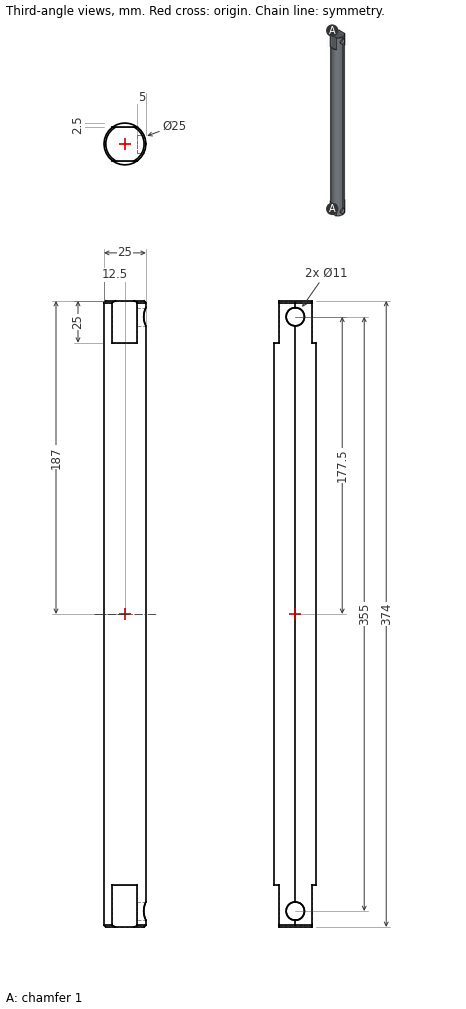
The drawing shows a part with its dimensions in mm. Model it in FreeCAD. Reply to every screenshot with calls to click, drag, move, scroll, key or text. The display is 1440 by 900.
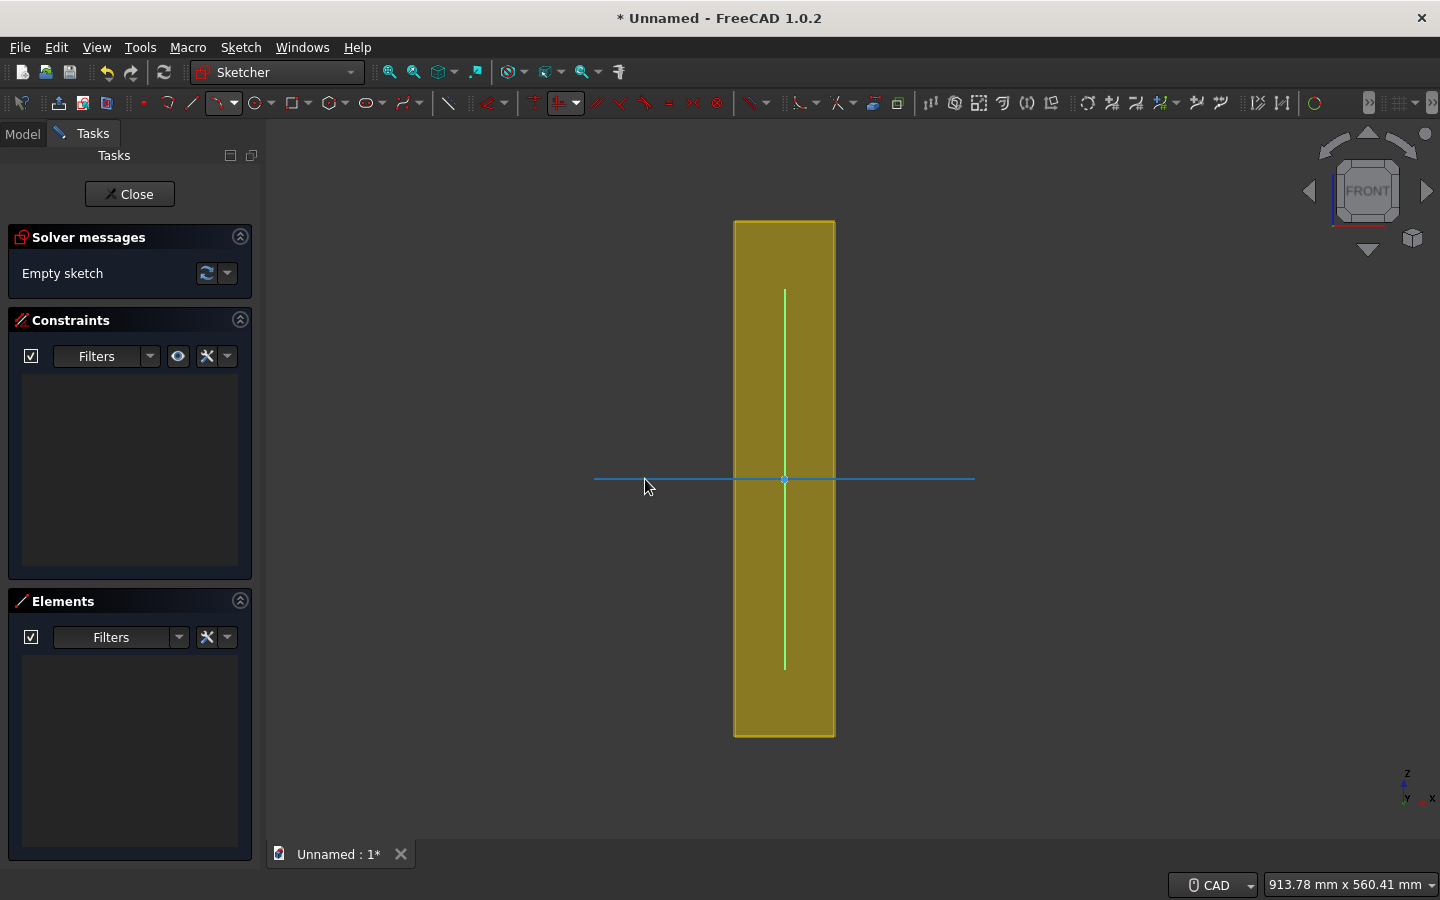
click(292, 104)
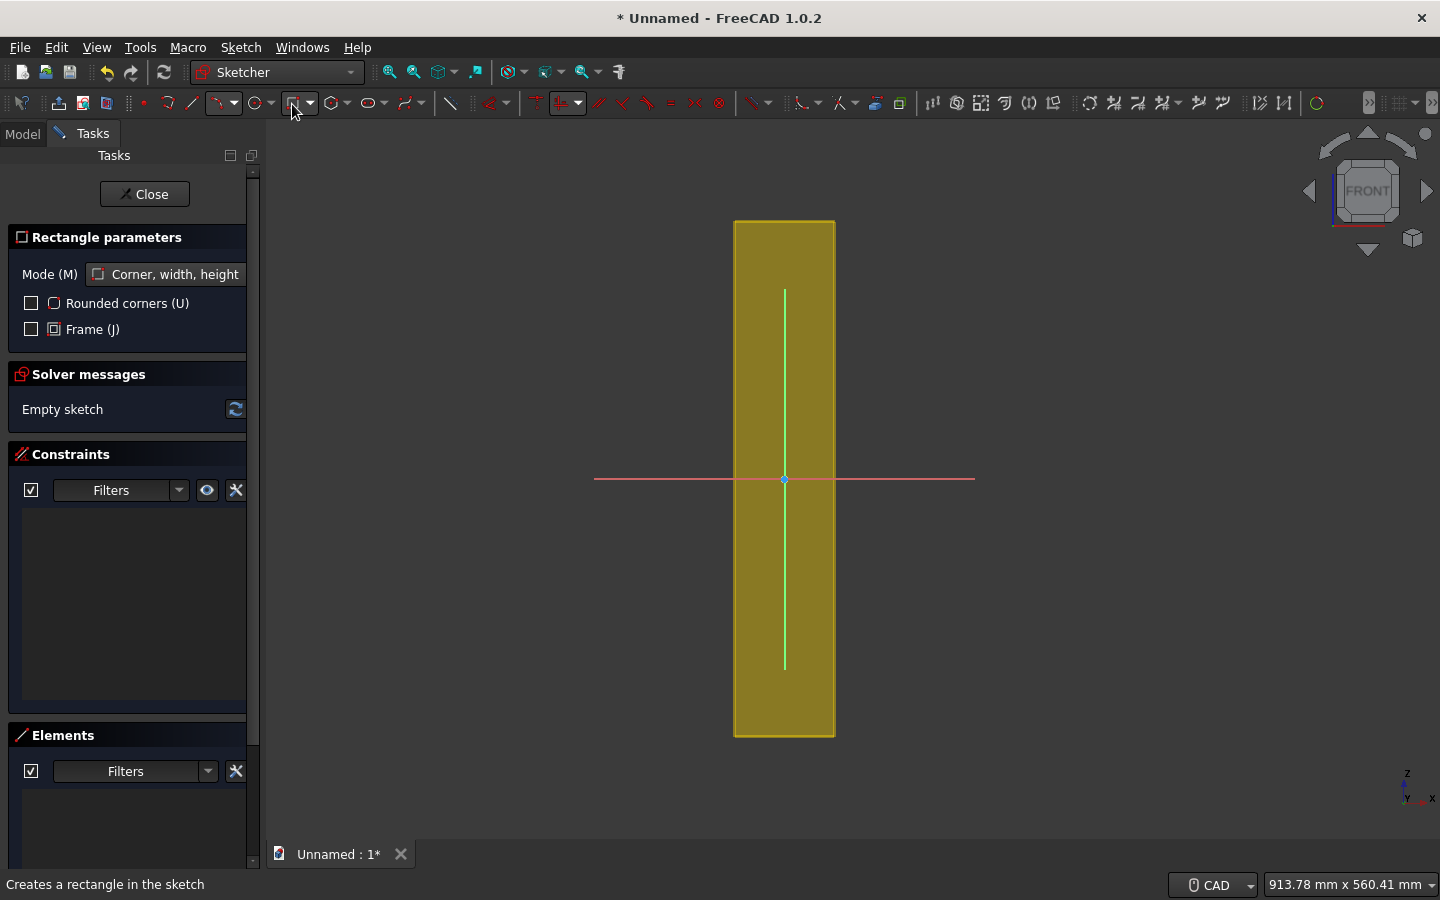
click(768, 239)
click(801, 271)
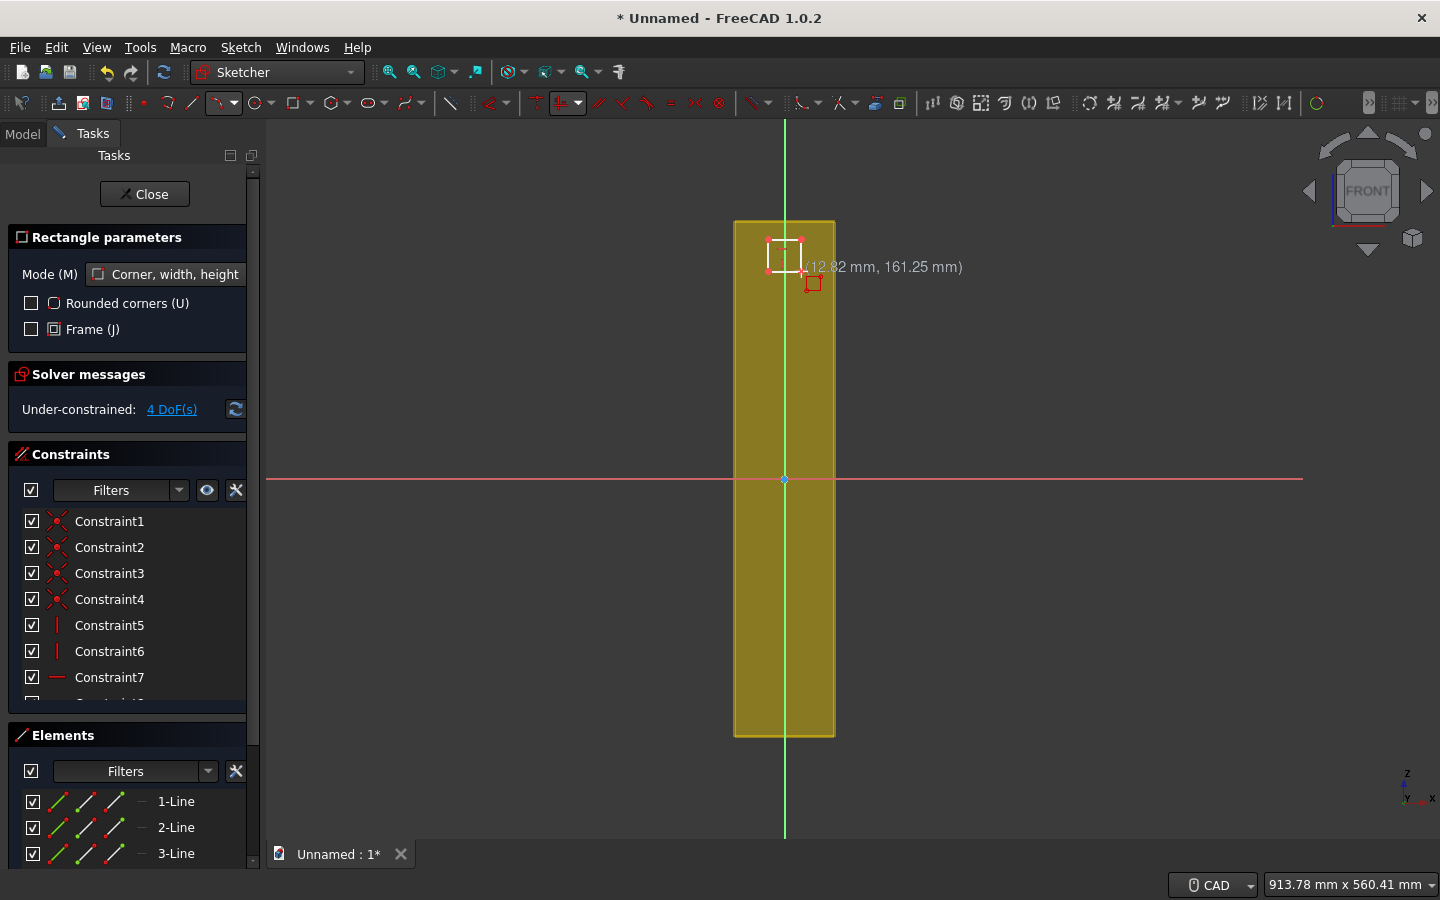
click(768, 687)
click(801, 719)
key(Escape)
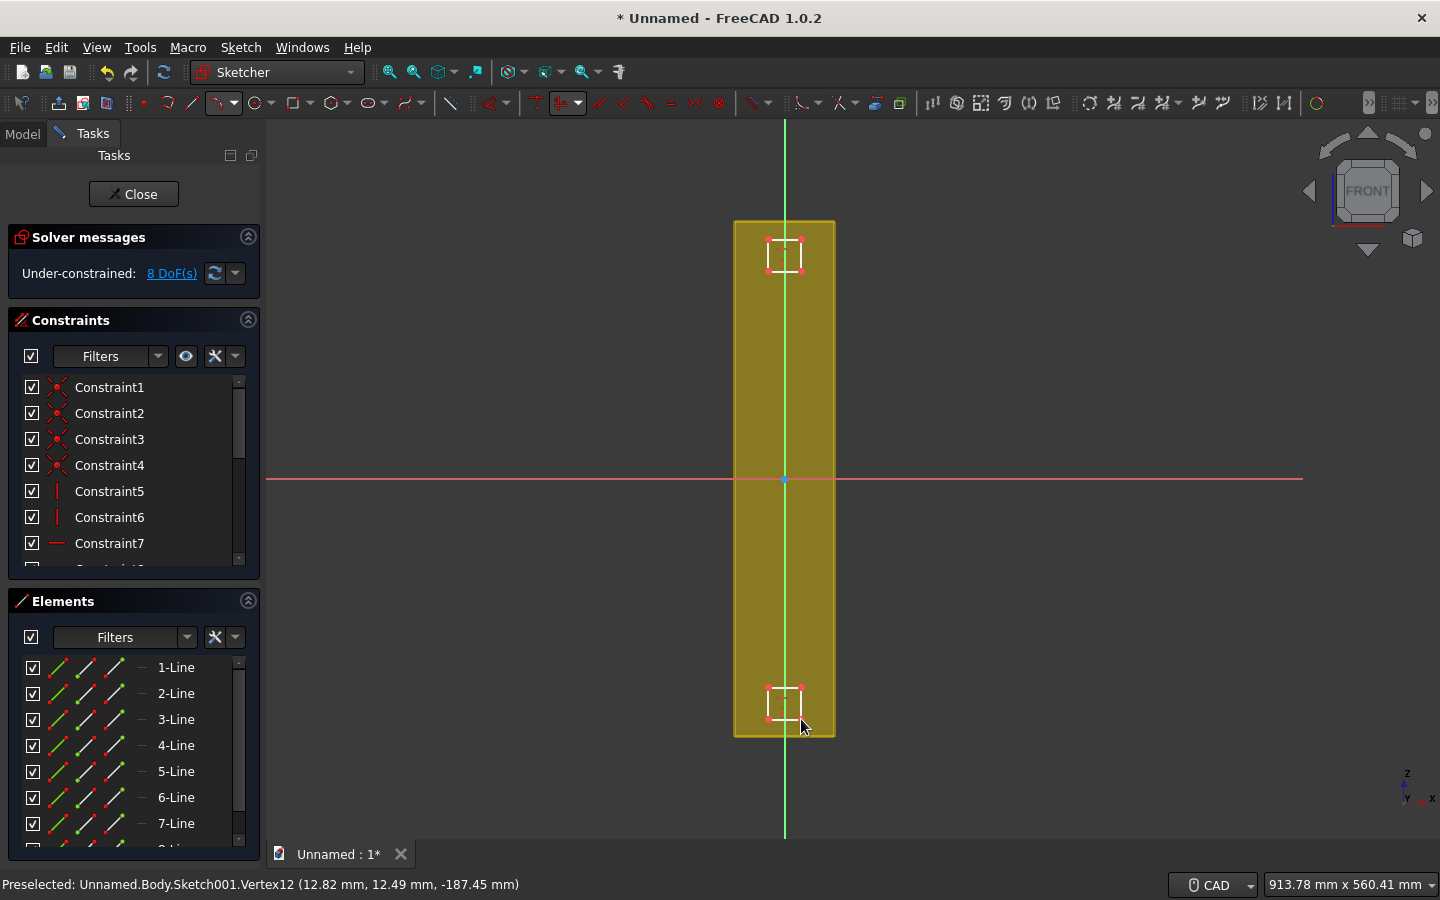
click(768, 272)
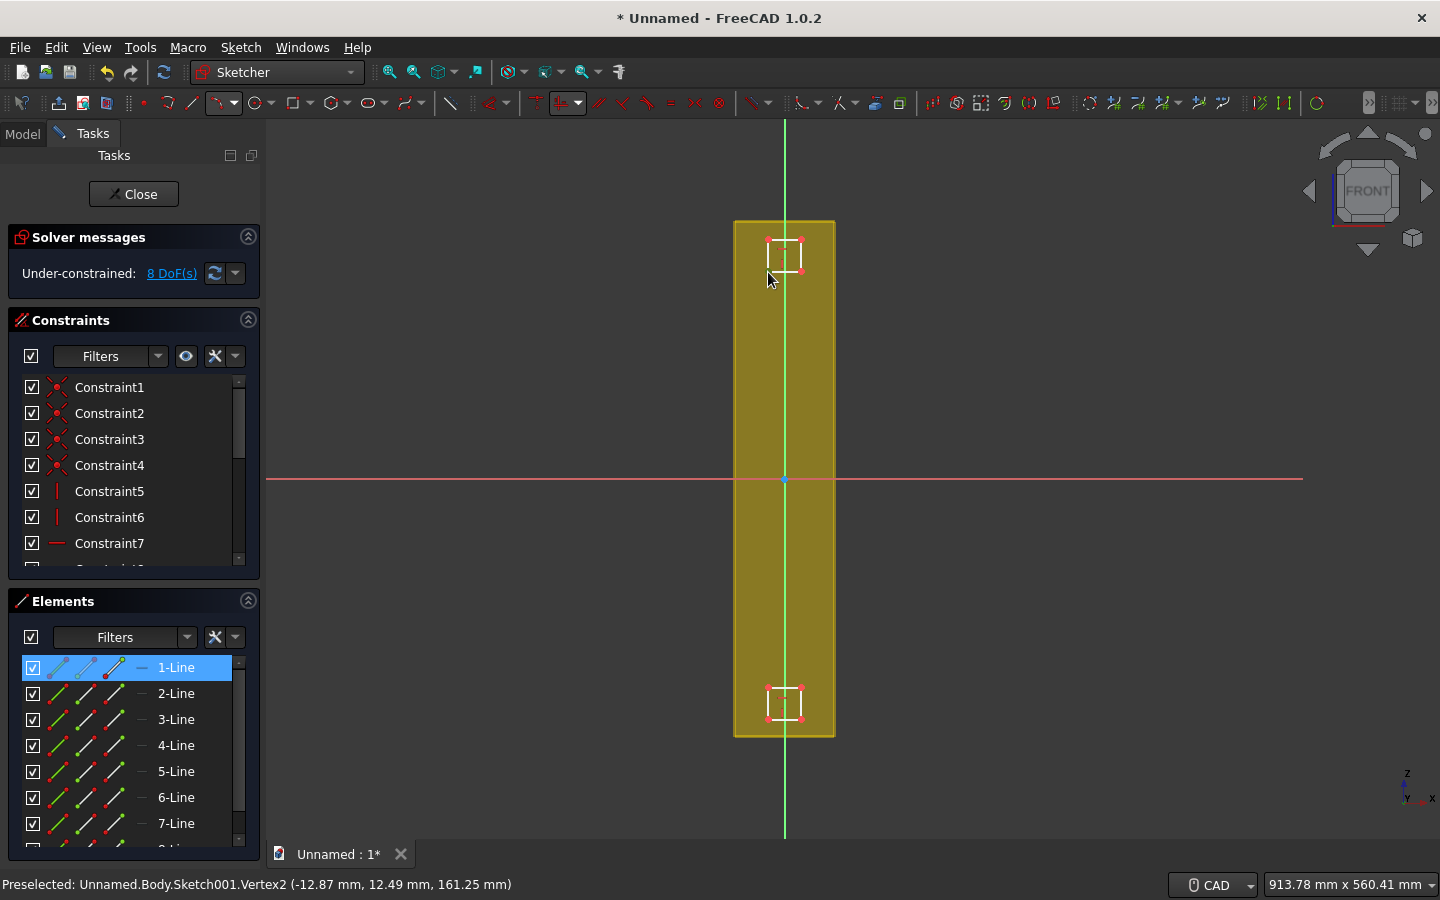
click(768, 688)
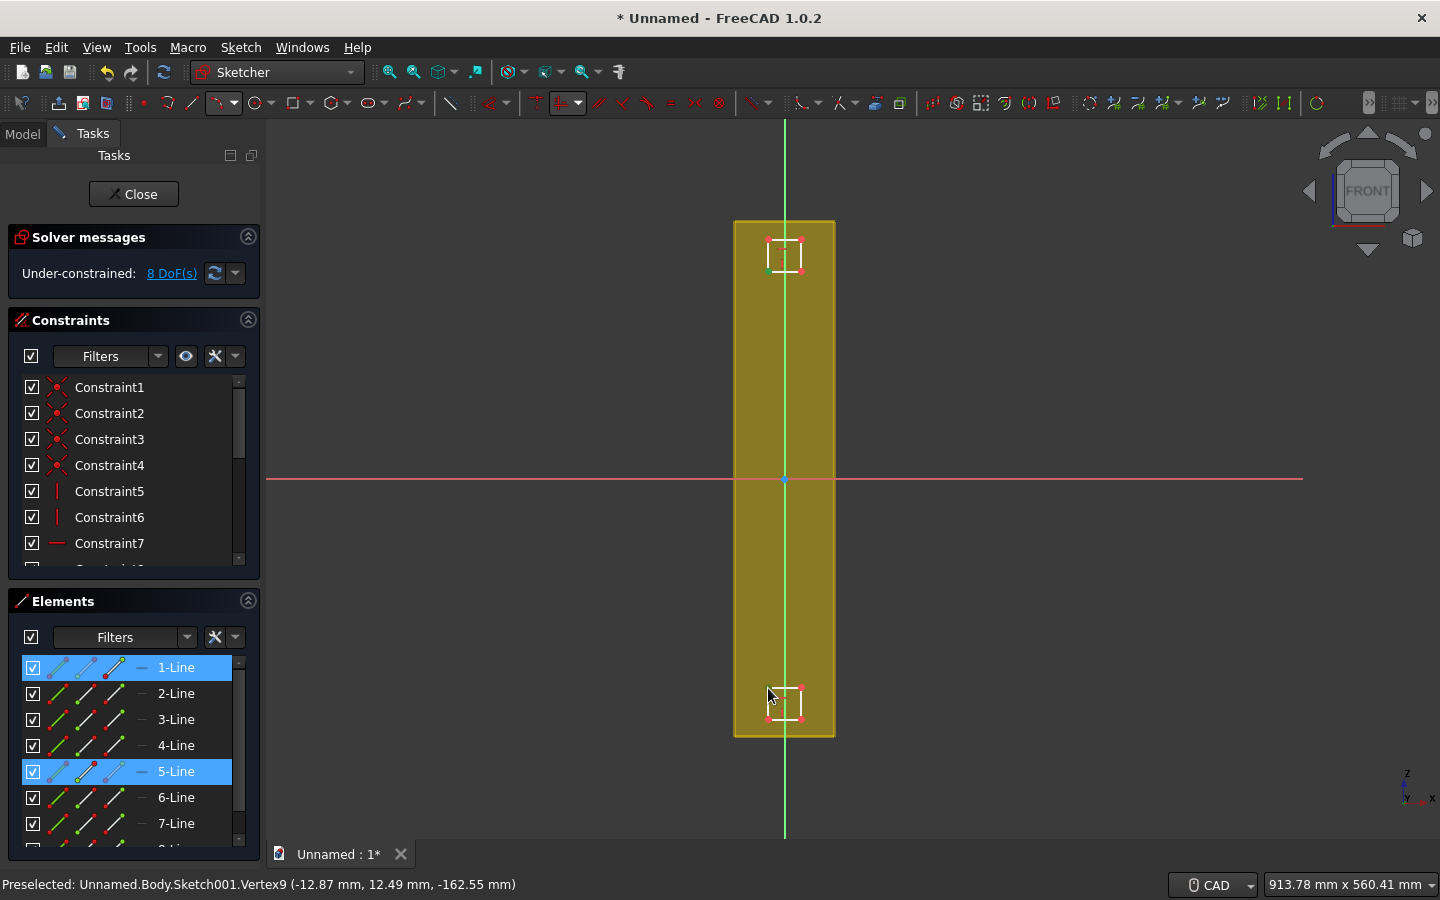
click(364, 479)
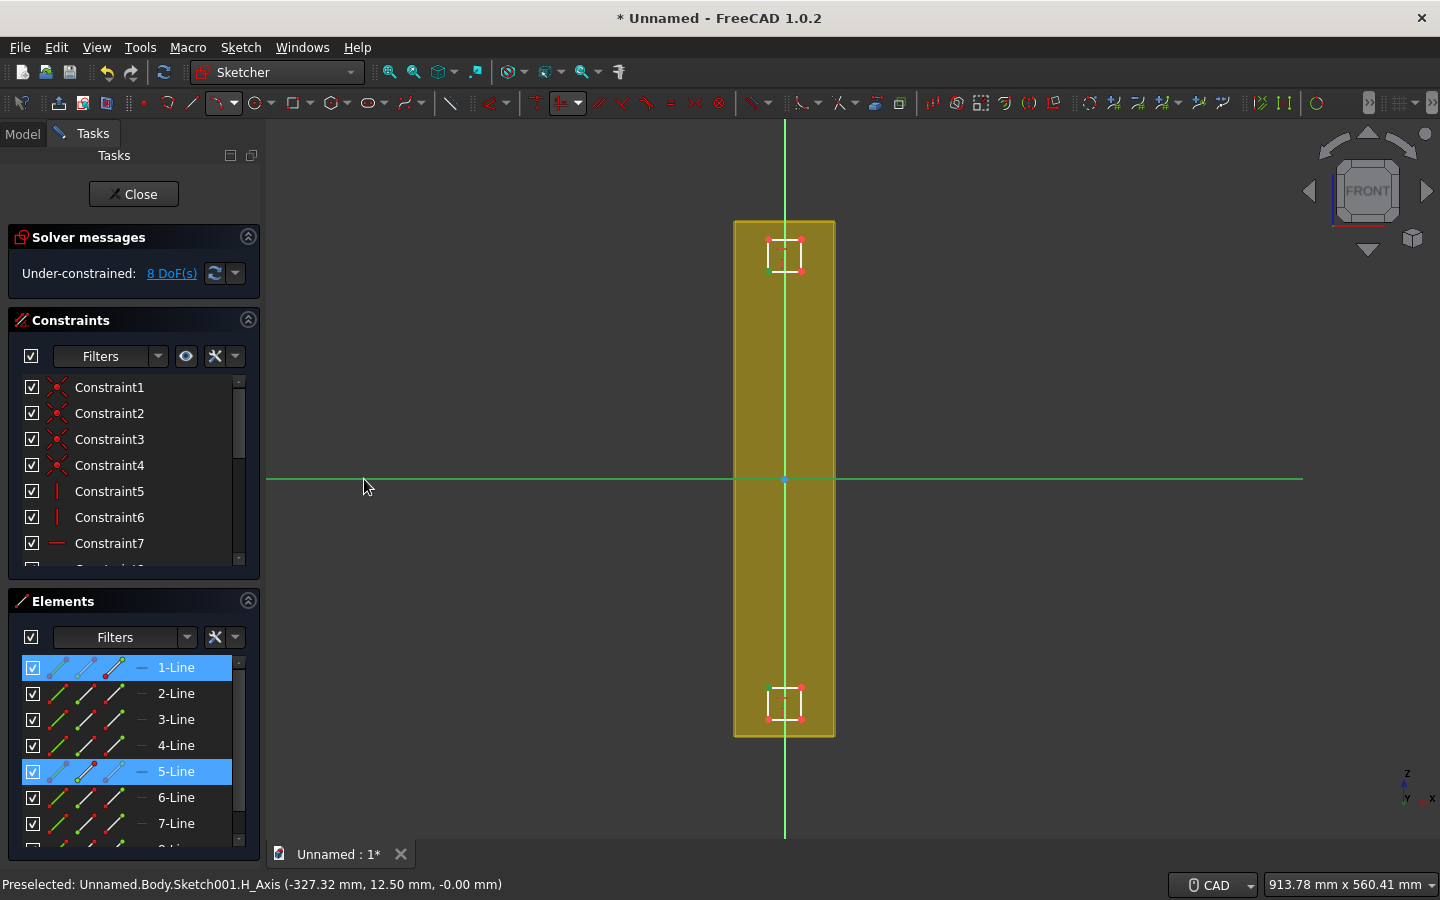
click(696, 104)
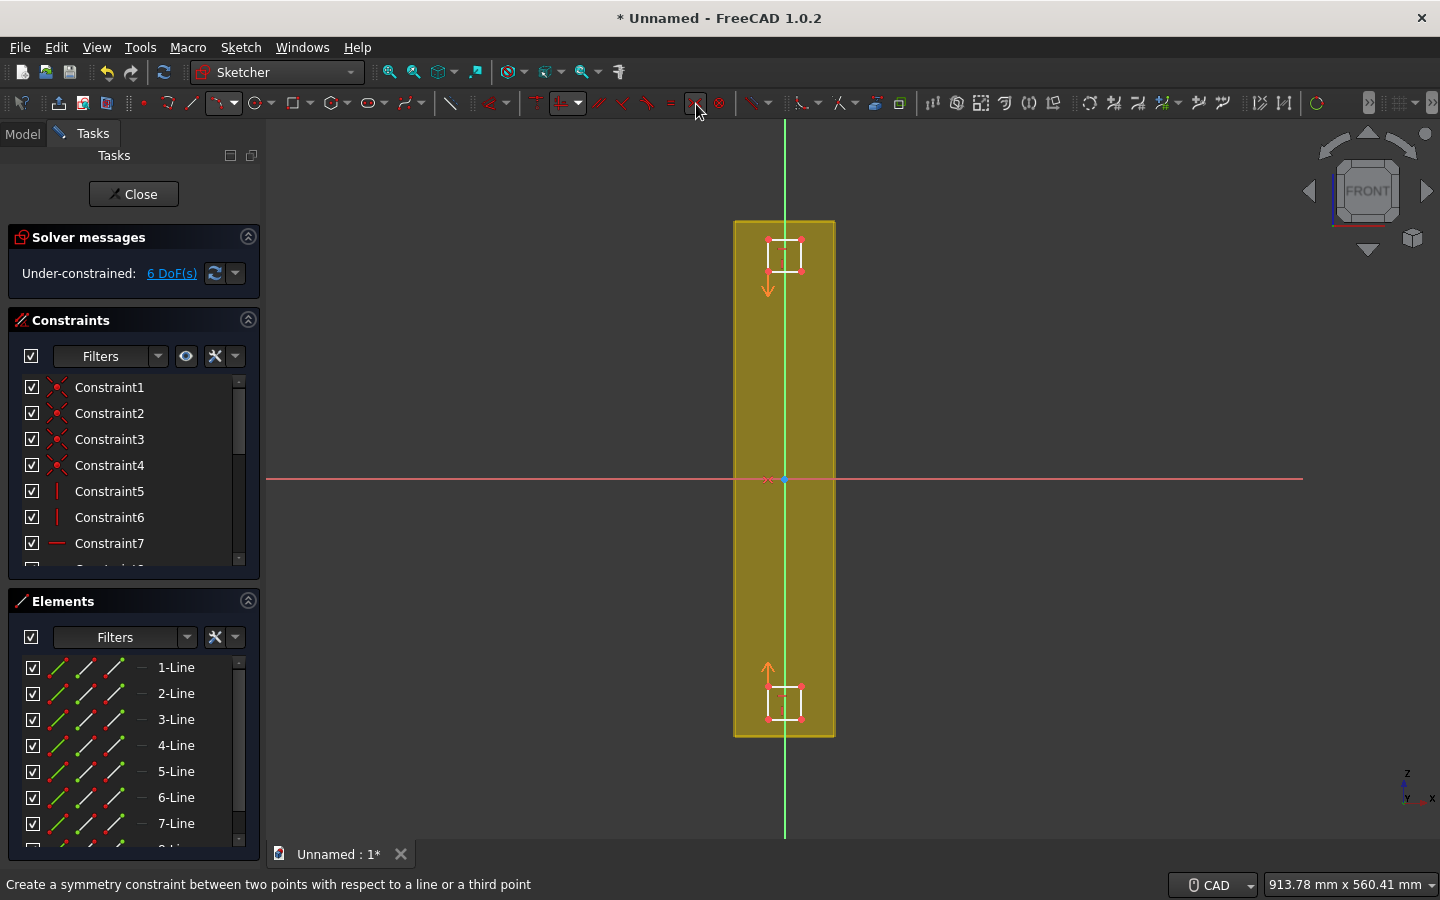
click(801, 240)